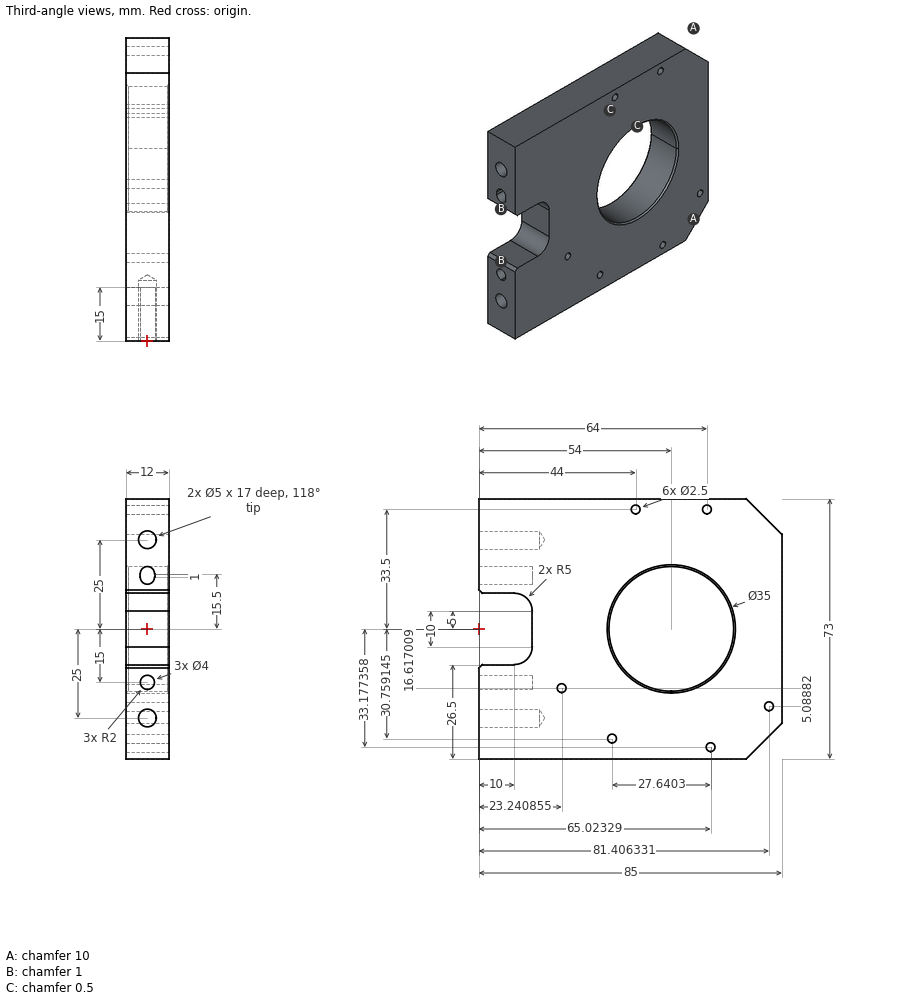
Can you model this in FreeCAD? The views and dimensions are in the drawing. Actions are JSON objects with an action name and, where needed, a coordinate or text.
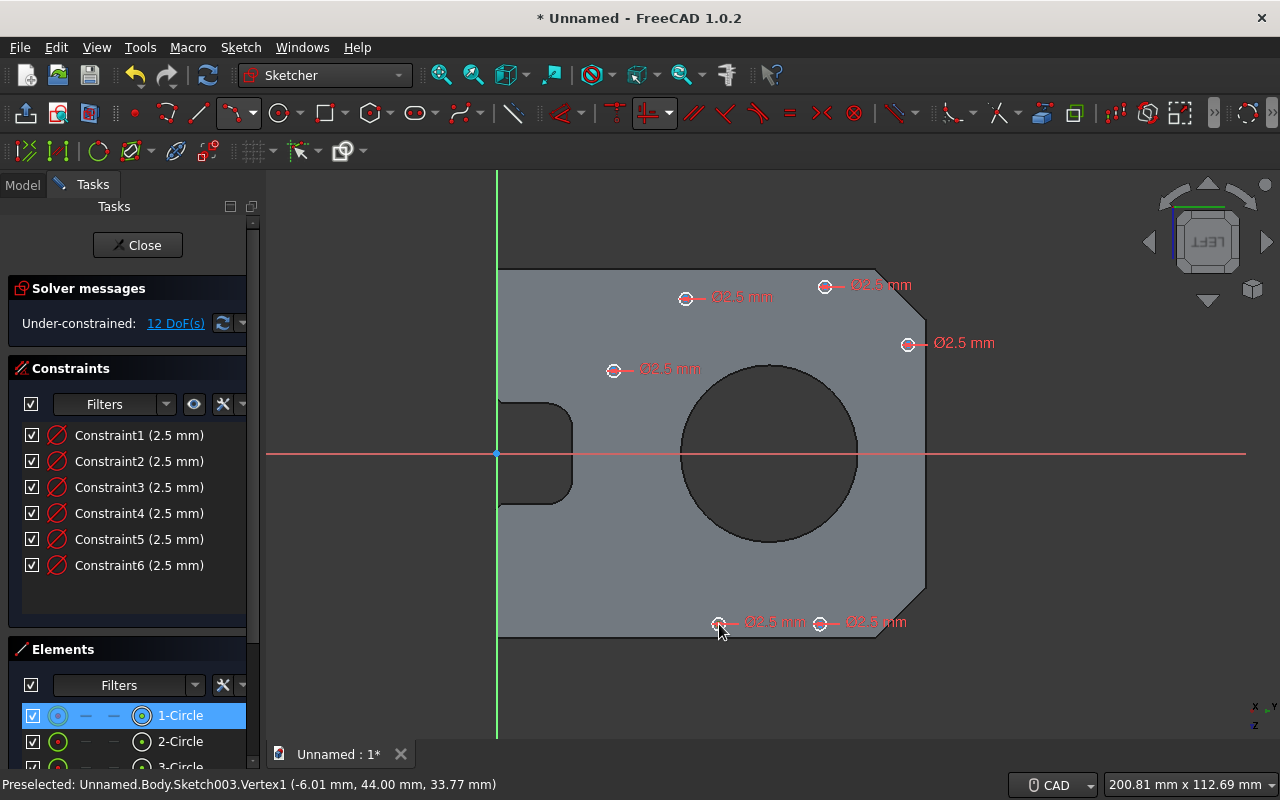
{"action": "left_click", "coordinate": [820, 624]}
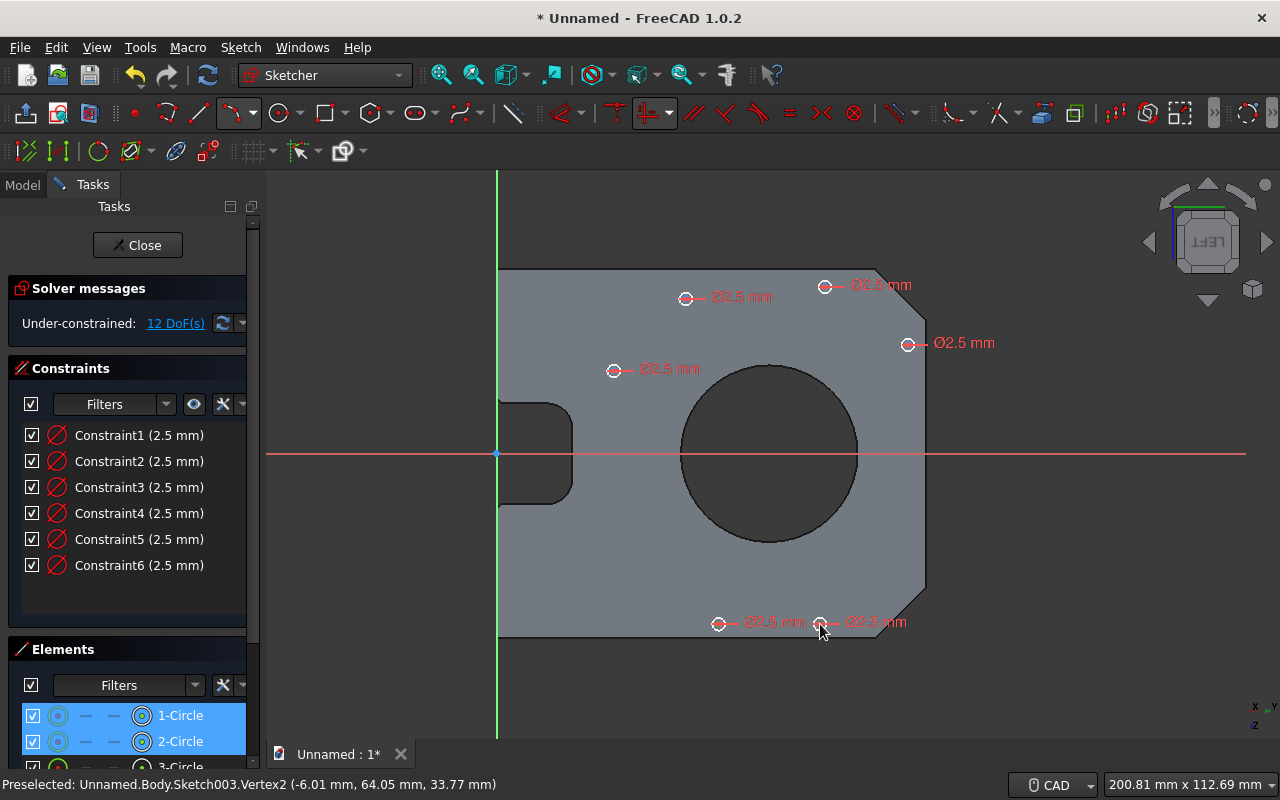
{"action": "left_click", "coordinate": [672, 114]}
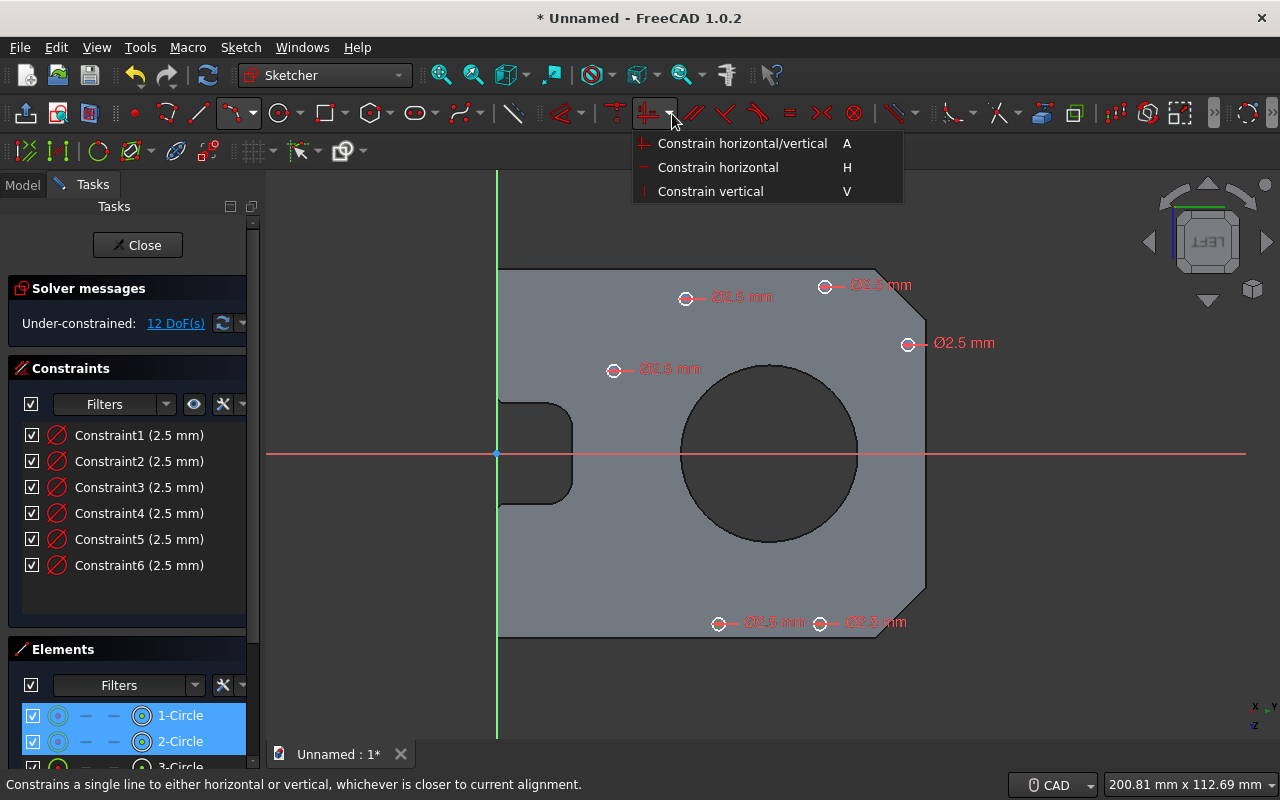
{"action": "left_click", "coordinate": [768, 167]}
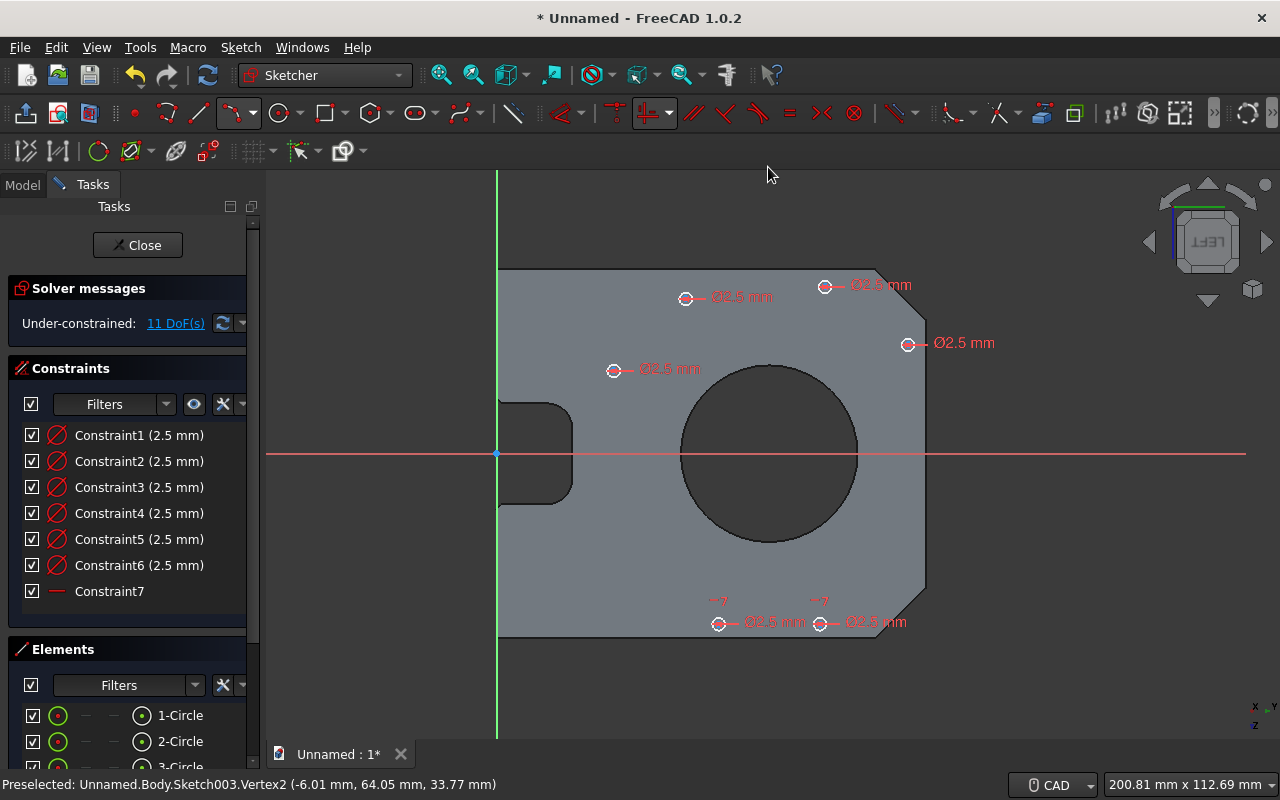
{"action": "left_click", "coordinate": [560, 114]}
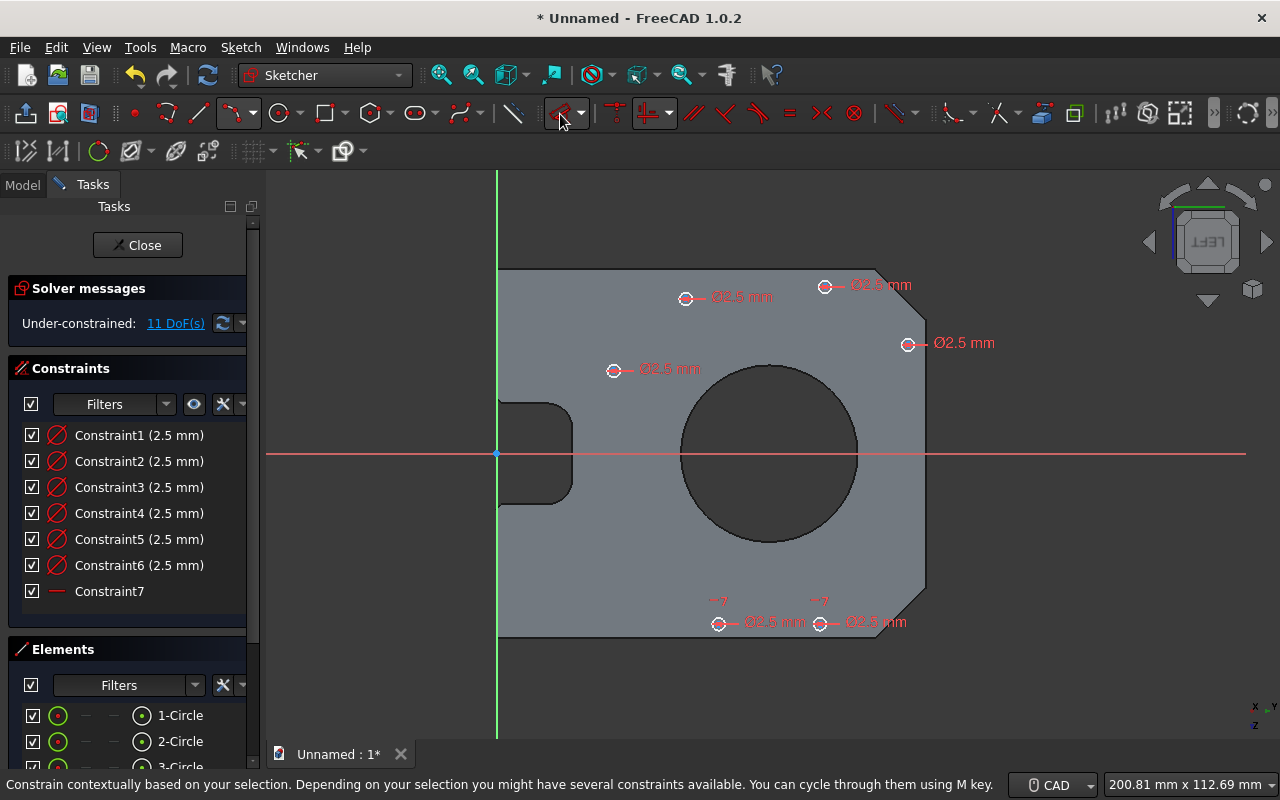
{"action": "left_click", "coordinate": [719, 624]}
{"action": "left_click", "coordinate": [608, 658]}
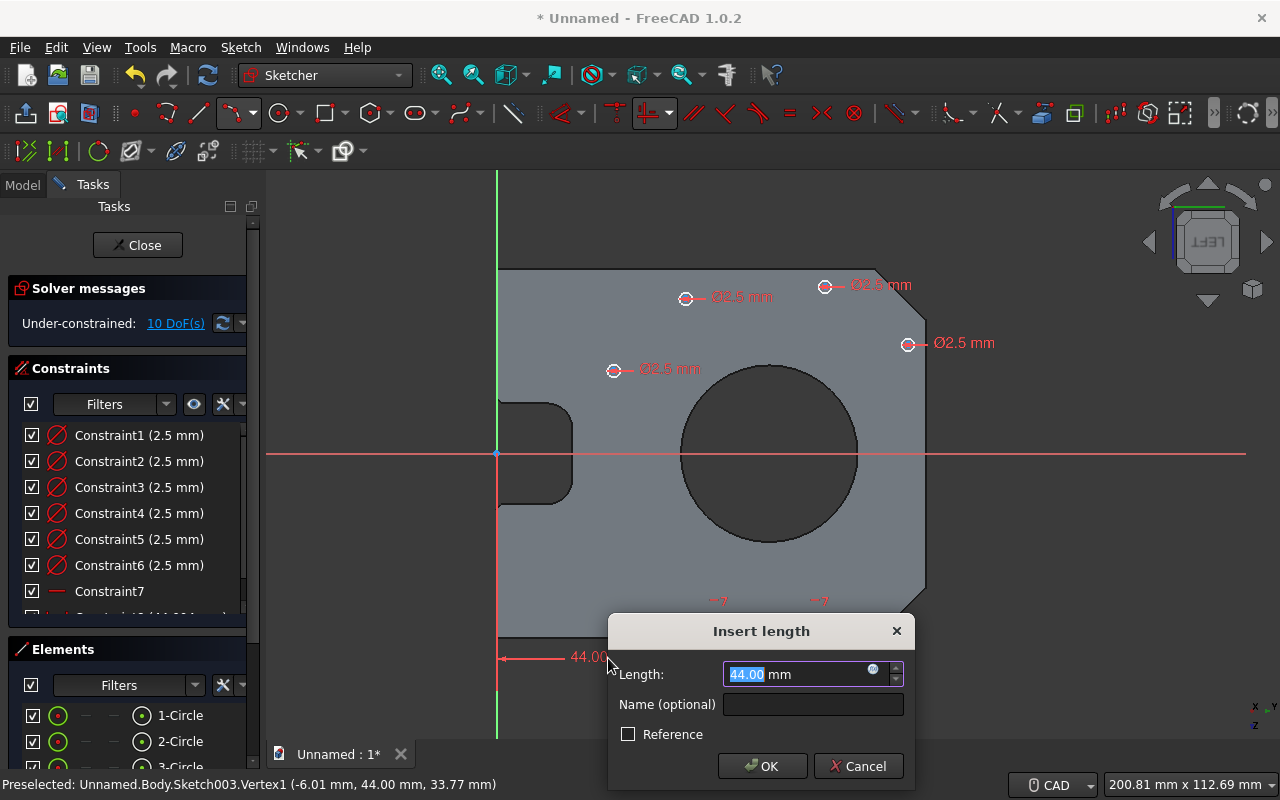
{"action": "type", "text": "44"}
{"action": "key", "text": "Return"}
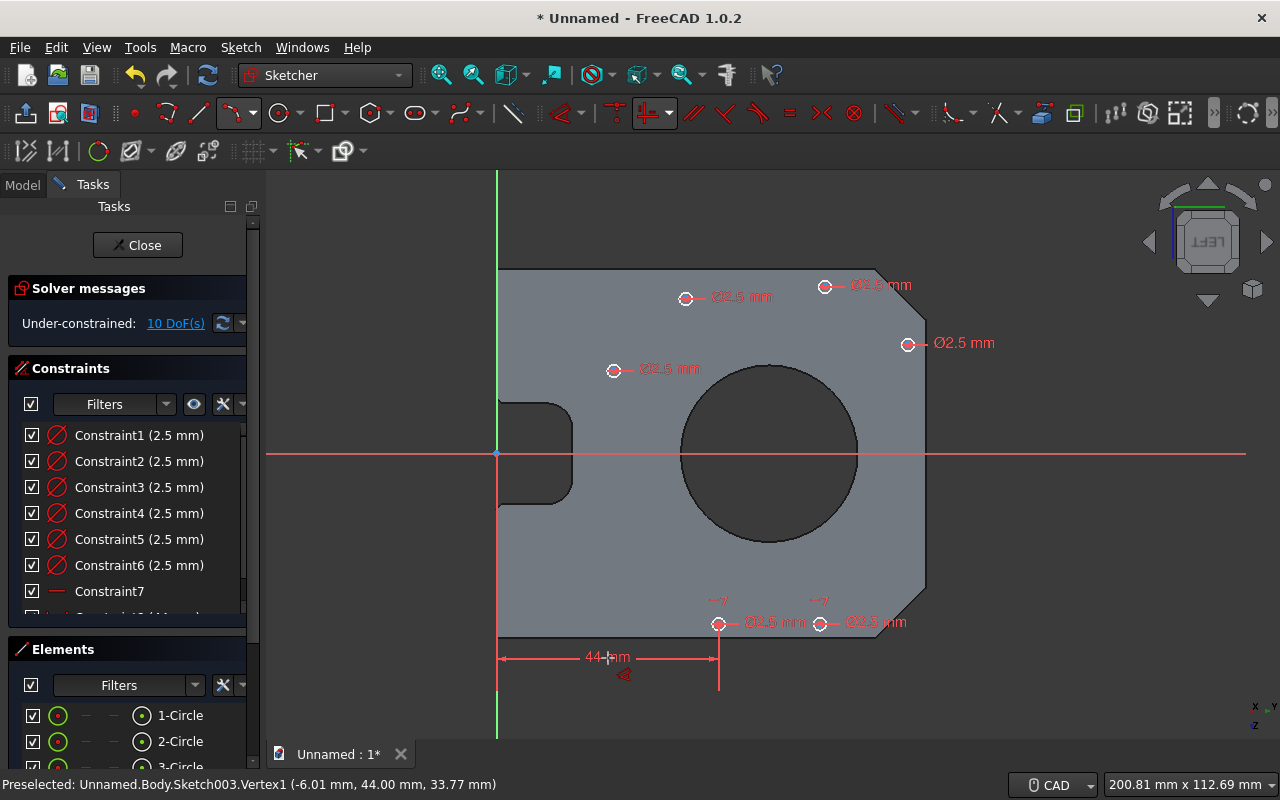
{"action": "left_click", "coordinate": [820, 624]}
{"action": "left_click", "coordinate": [733, 658]}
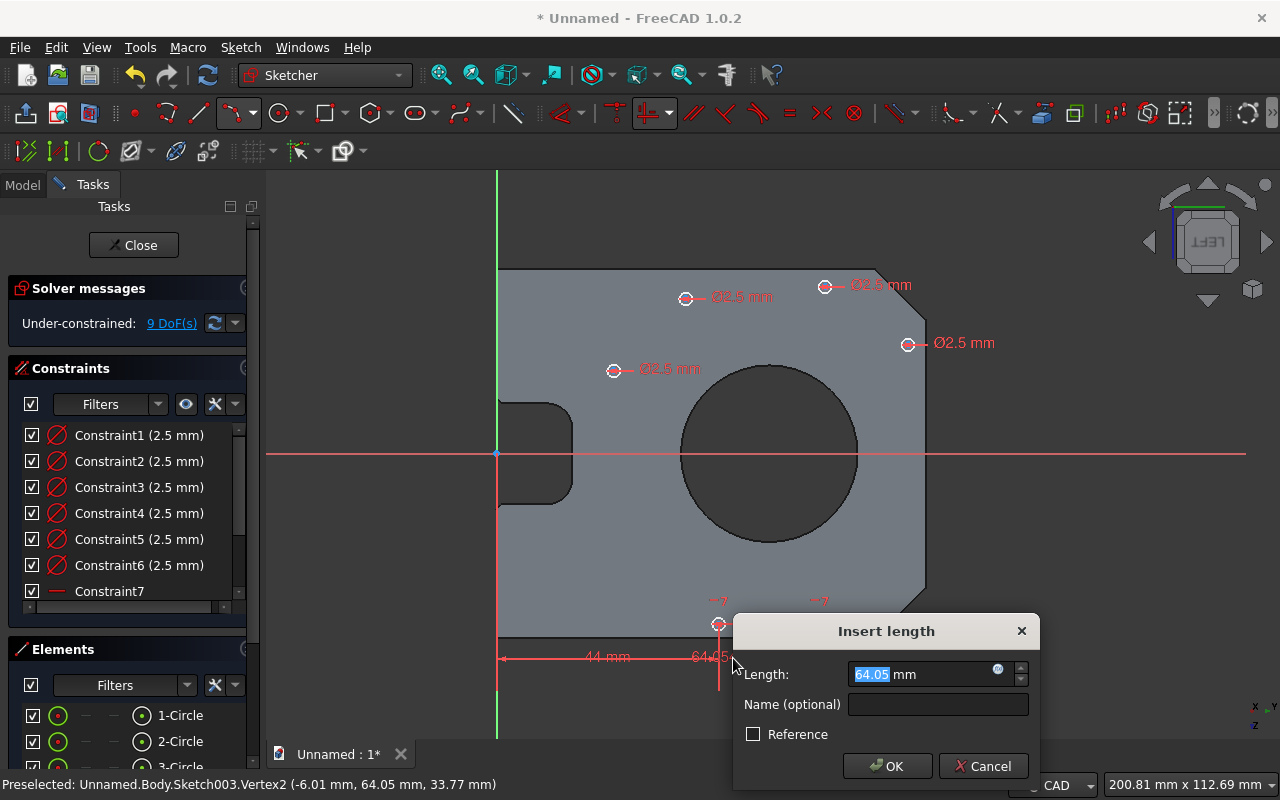
{"action": "type", "text": "64"}
{"action": "key", "text": "Return"}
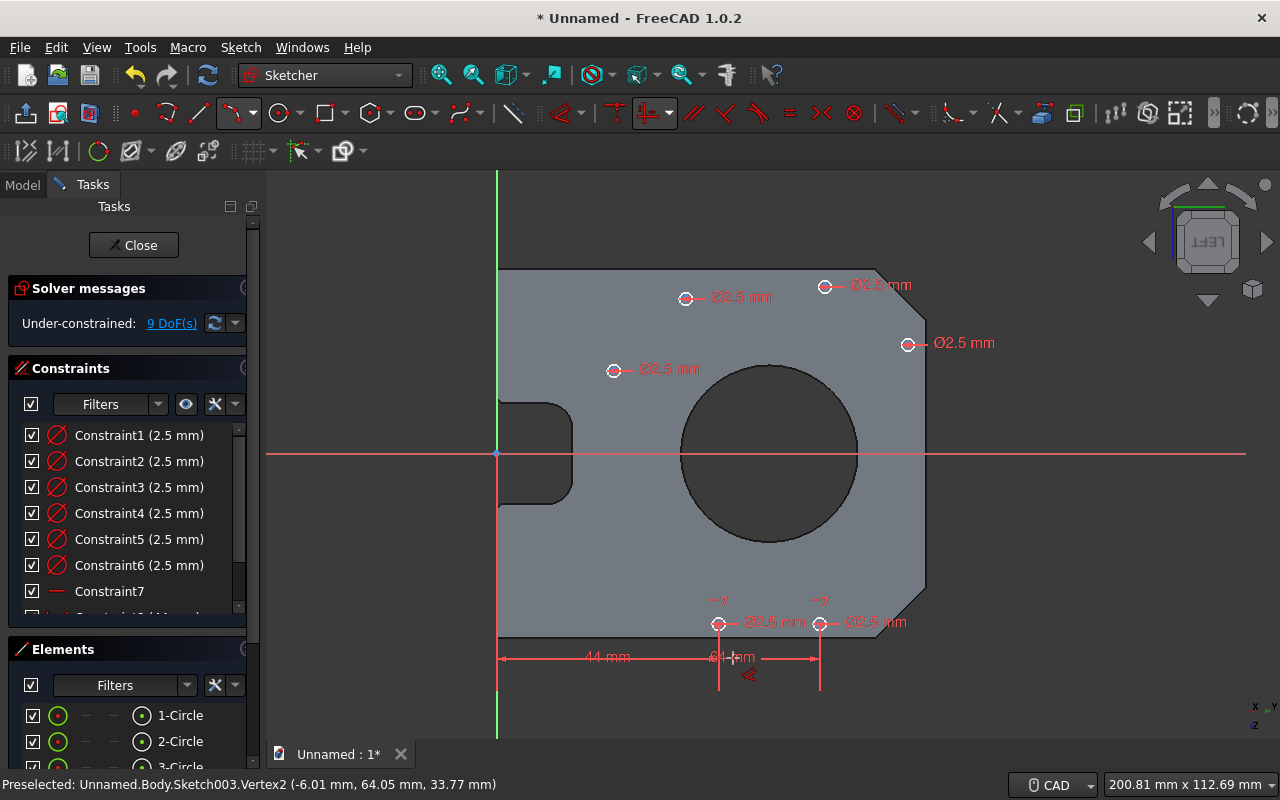
{"action": "left_click", "coordinate": [719, 624]}
{"action": "left_click", "coordinate": [463, 539]}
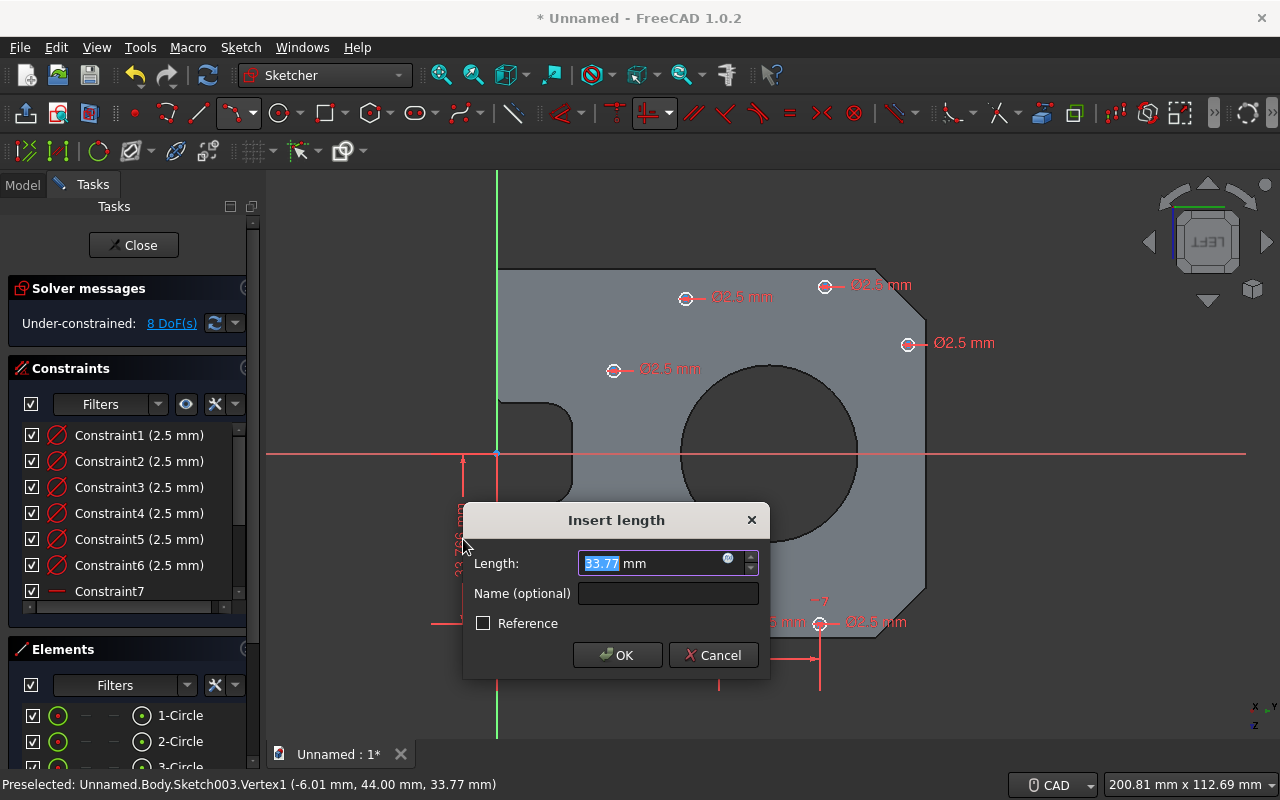
{"action": "type", "text": "33.5"}
{"action": "key", "text": "Return"}